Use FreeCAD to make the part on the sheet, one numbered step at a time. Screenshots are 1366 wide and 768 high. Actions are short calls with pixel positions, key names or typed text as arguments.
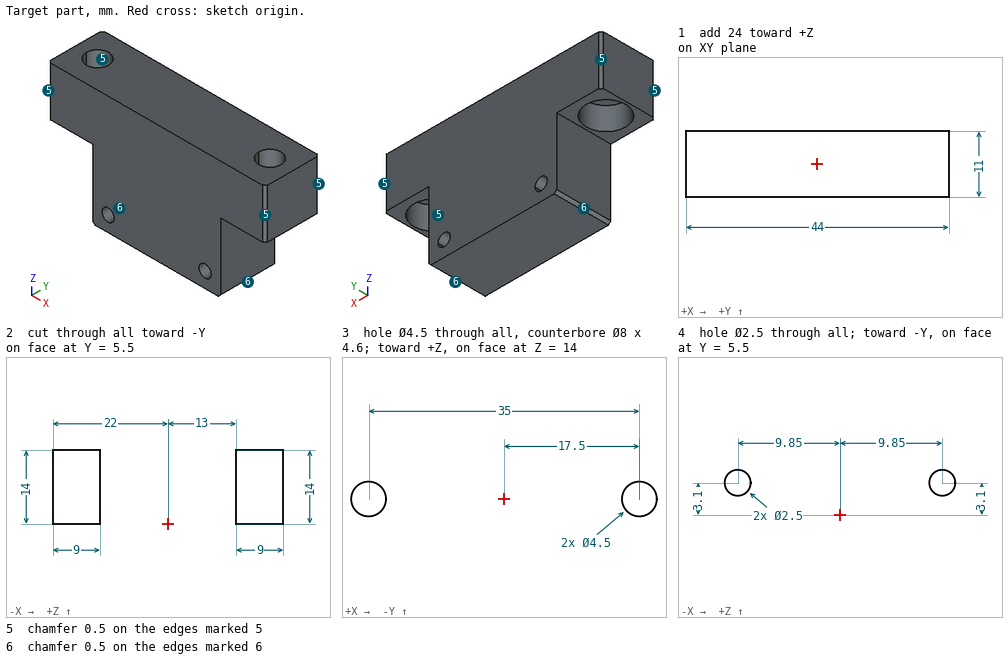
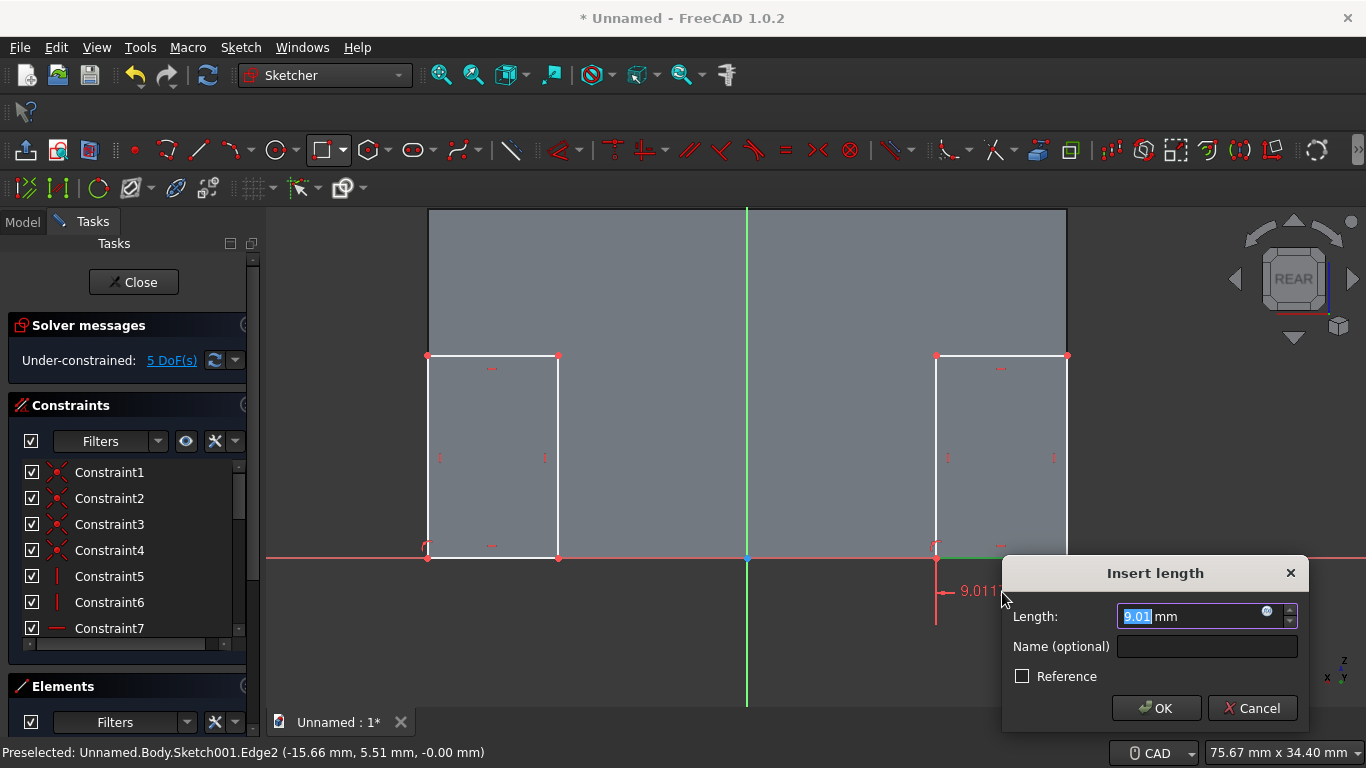
text(9)
key(Return)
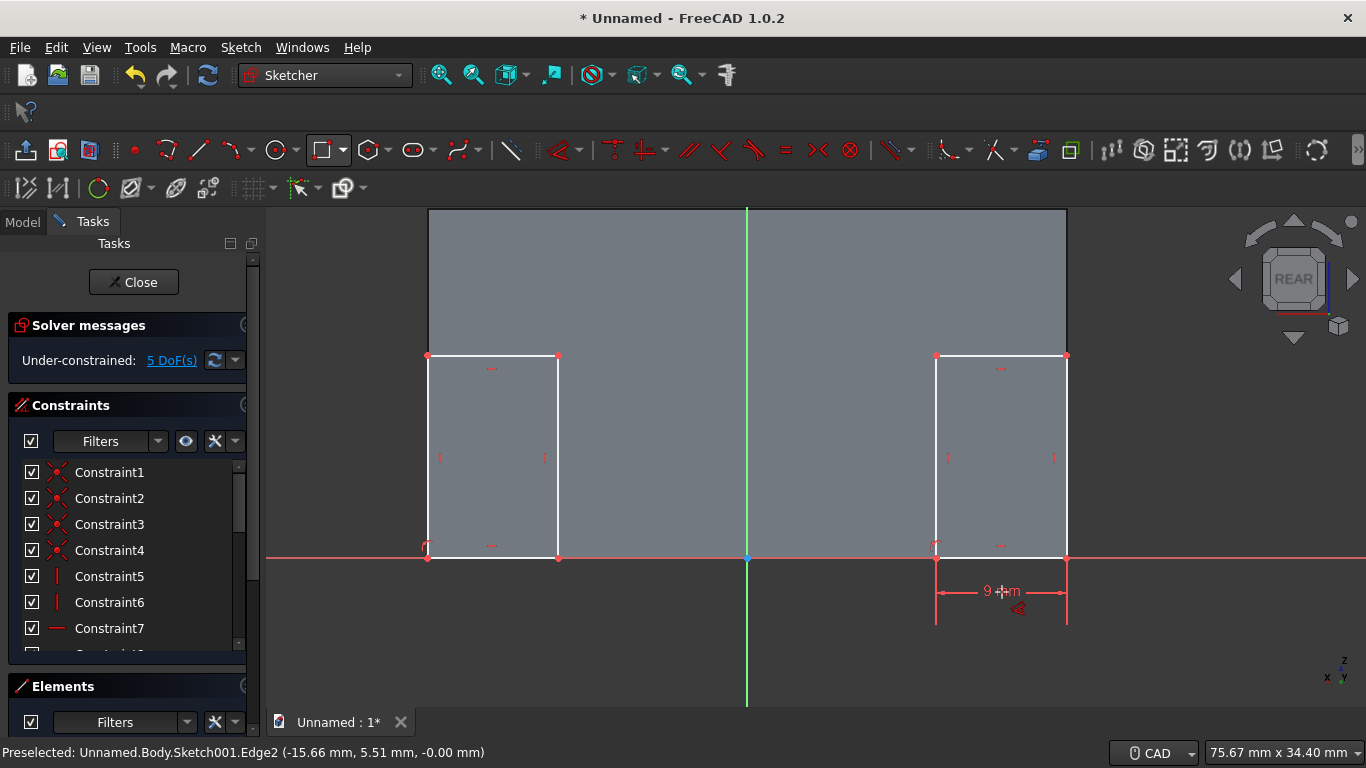
click(467, 558)
click(493, 592)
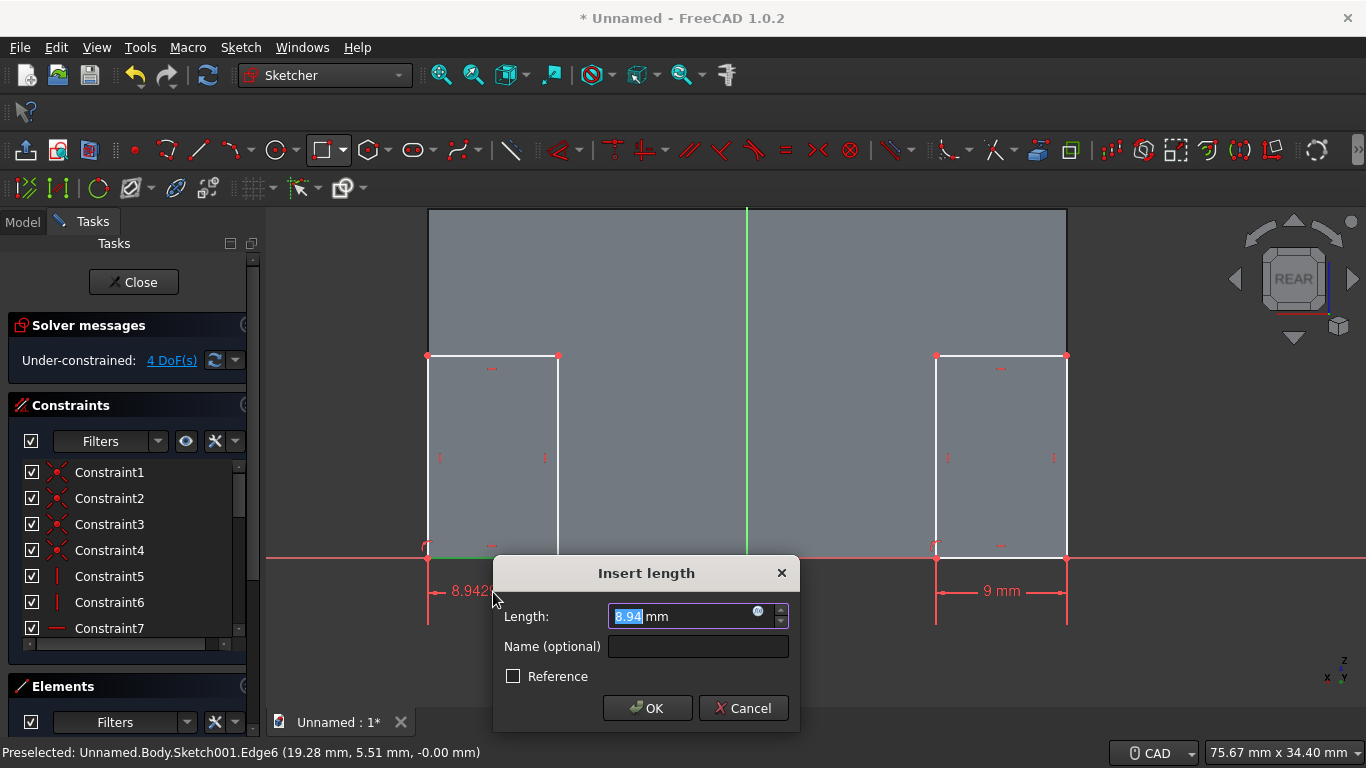
text(9)
key(Return)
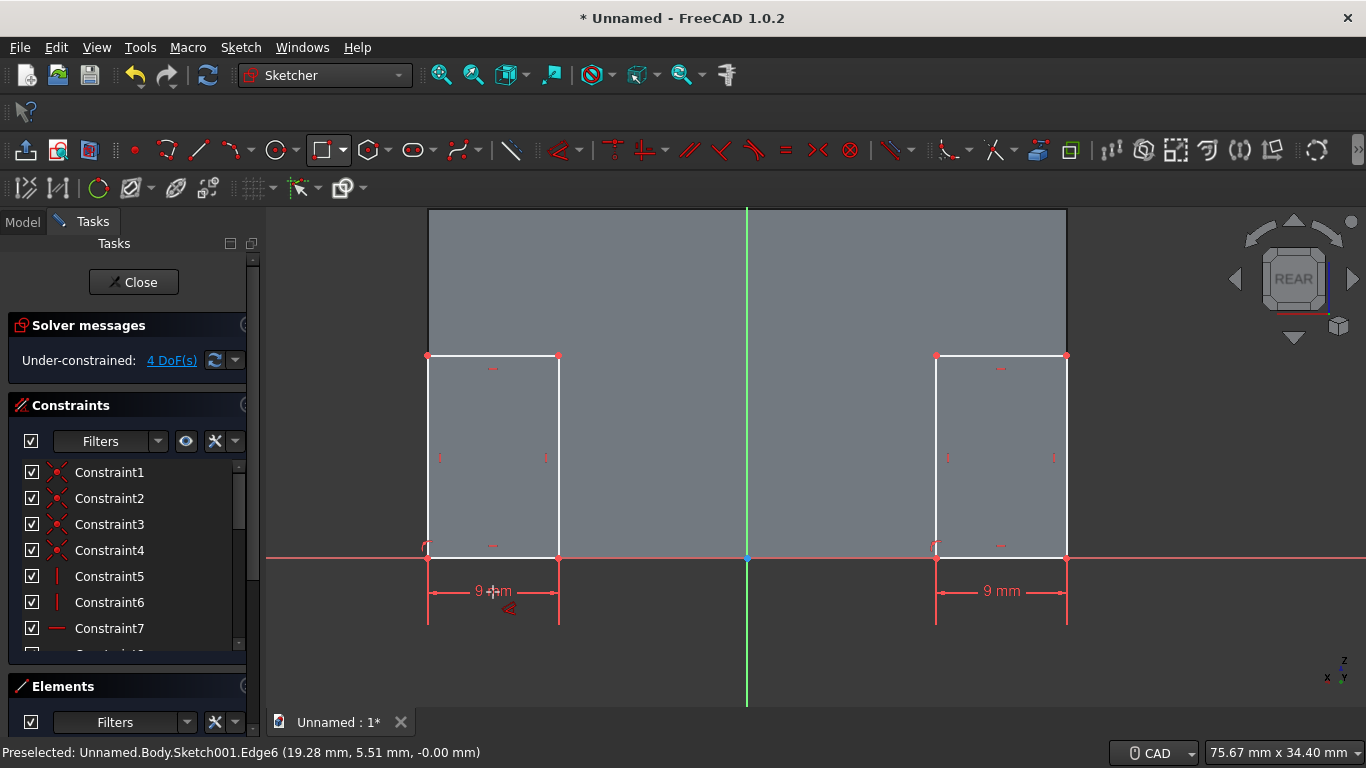
click(936, 417)
click(970, 457)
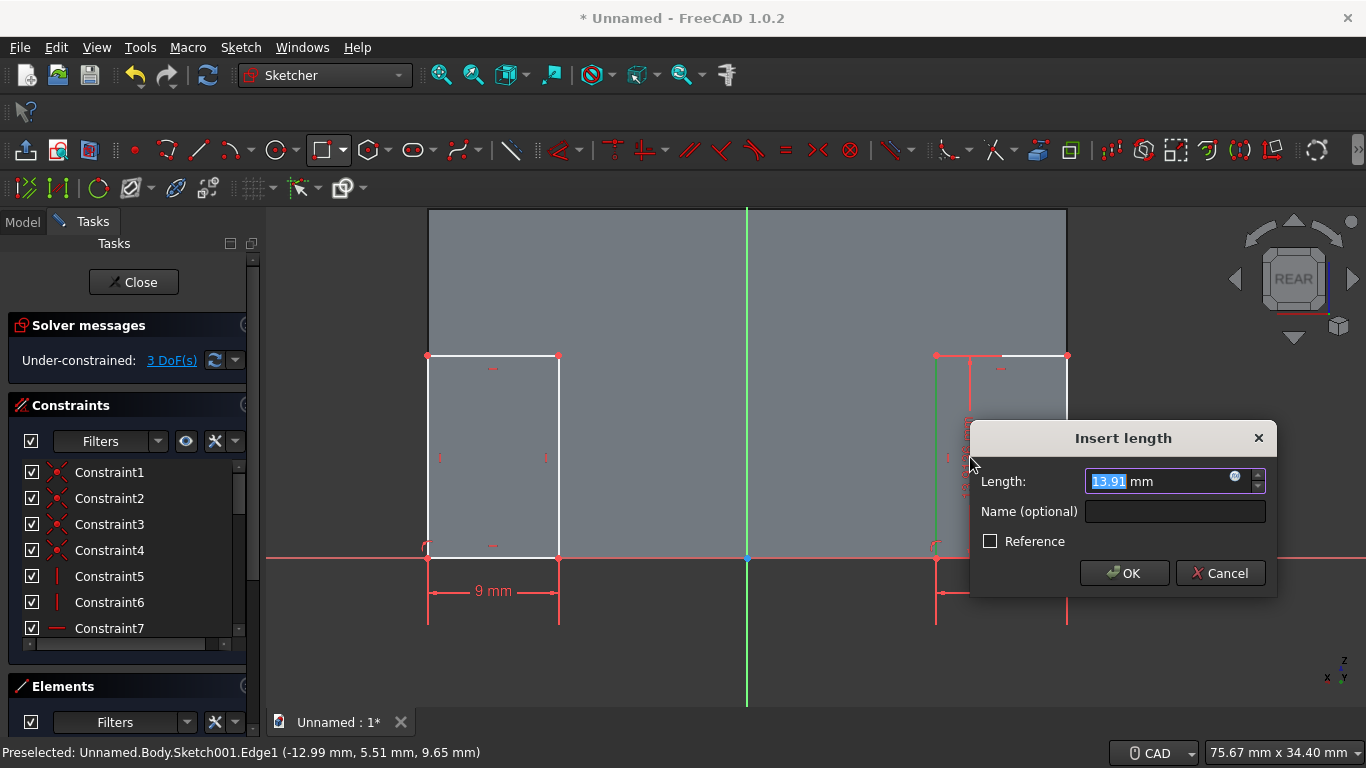
text(14)
key(Return)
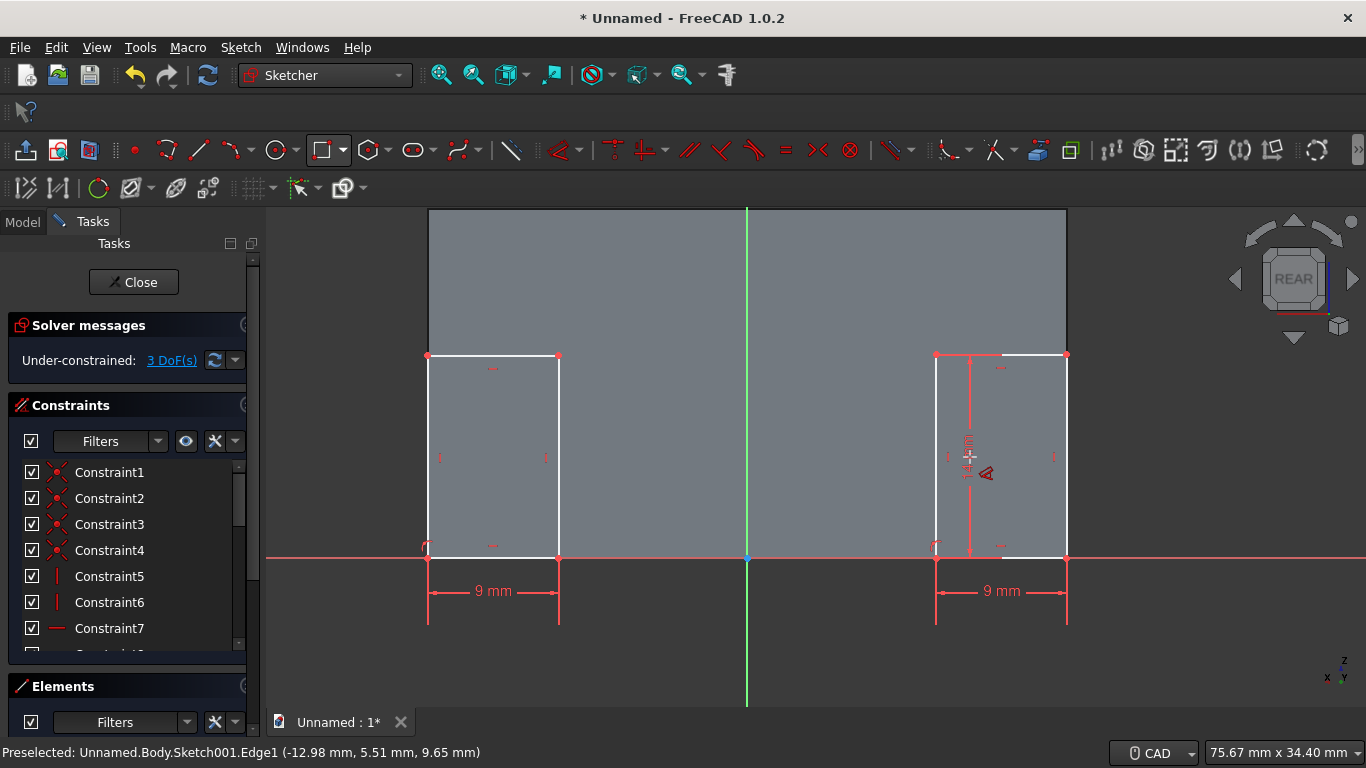
click(428, 417)
click(394, 457)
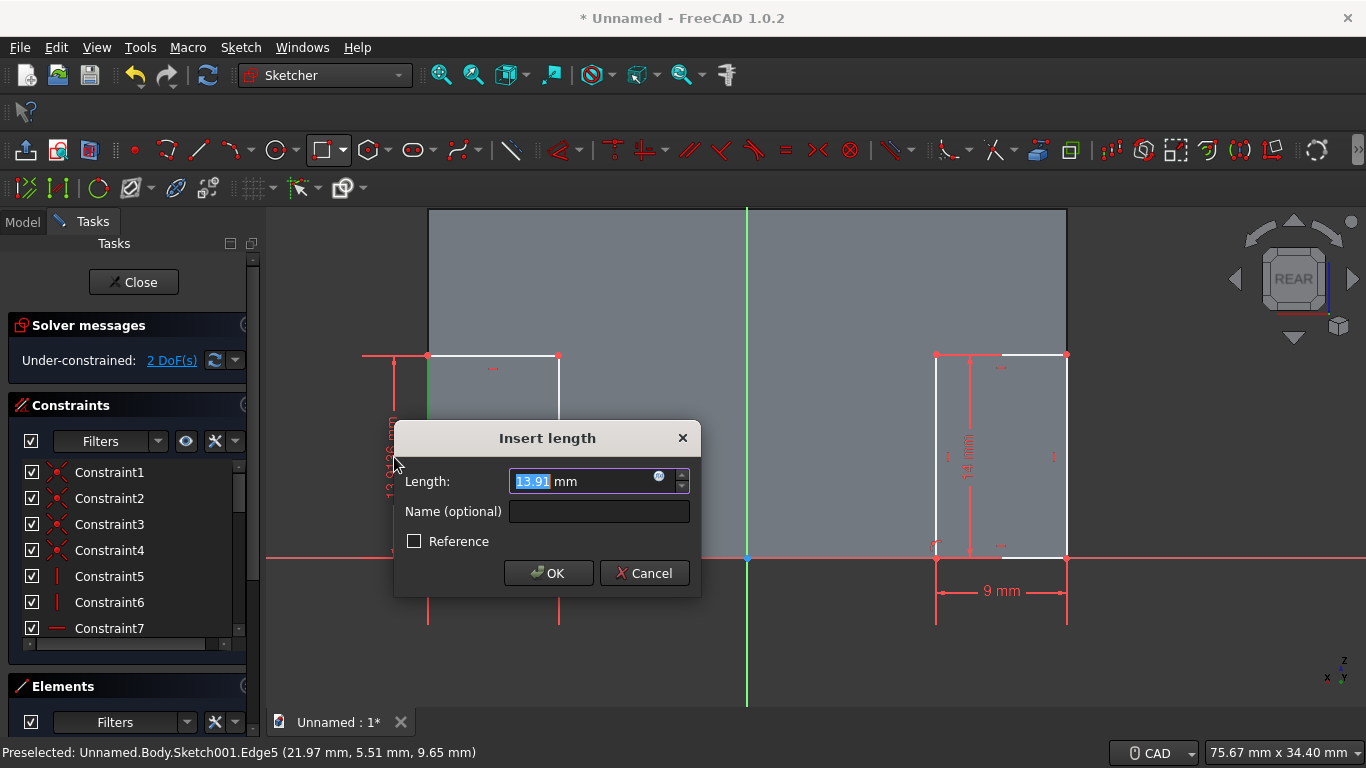
text(14)
key(Return)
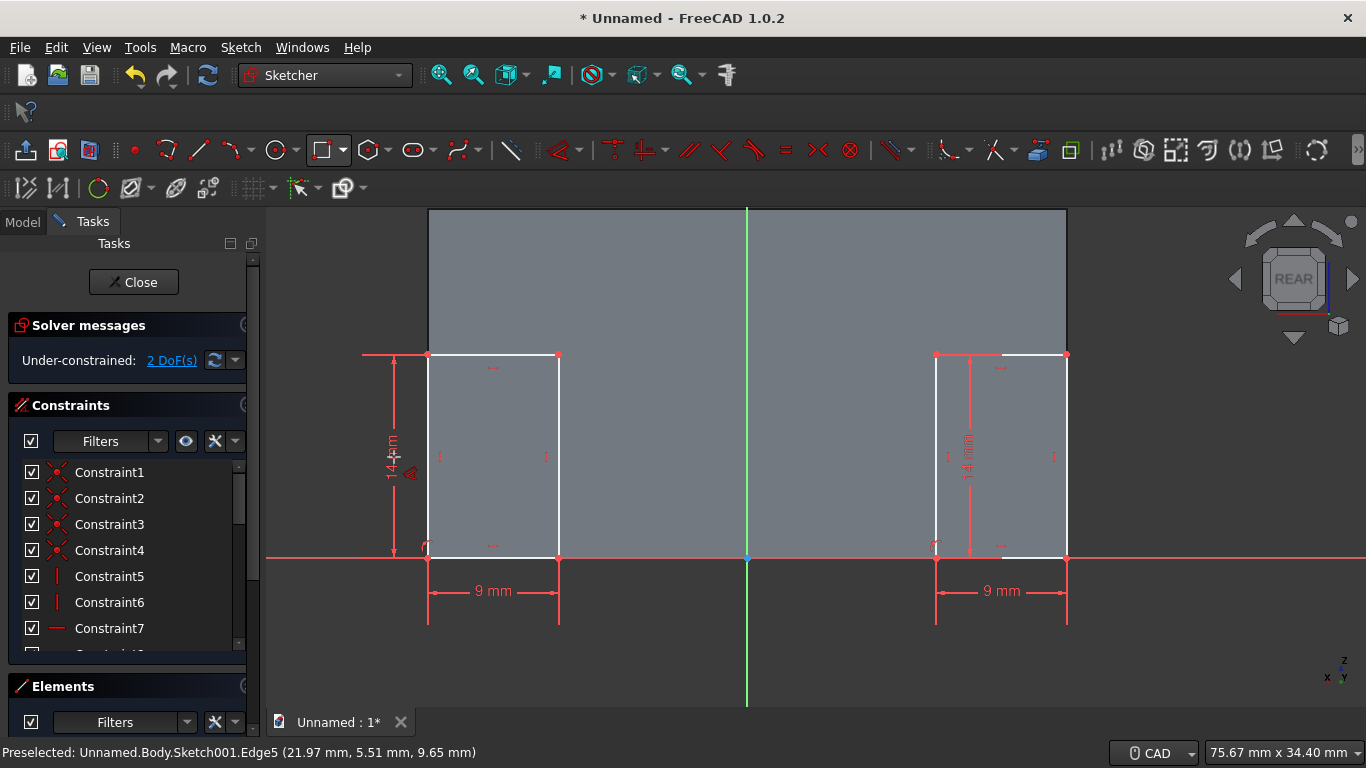
click(936, 355)
click(842, 592)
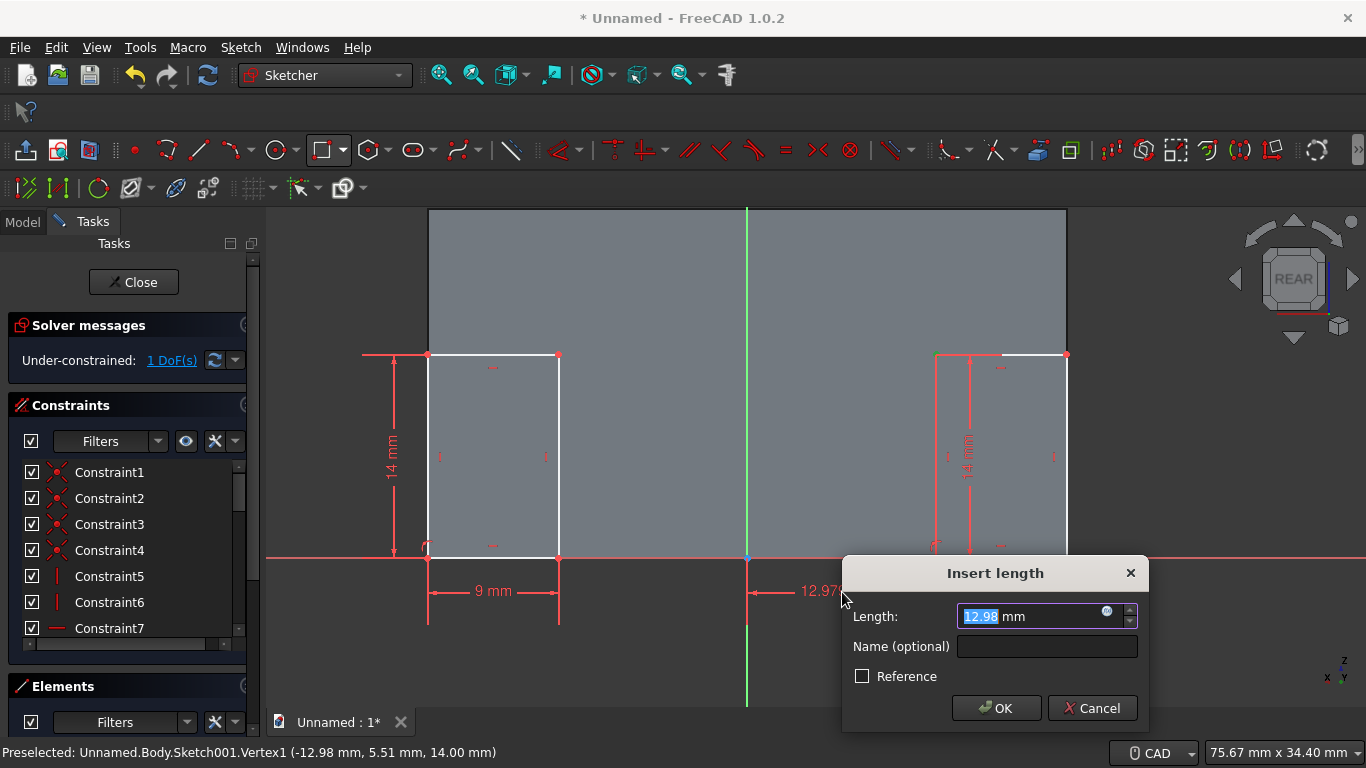
text(13)
key(Return)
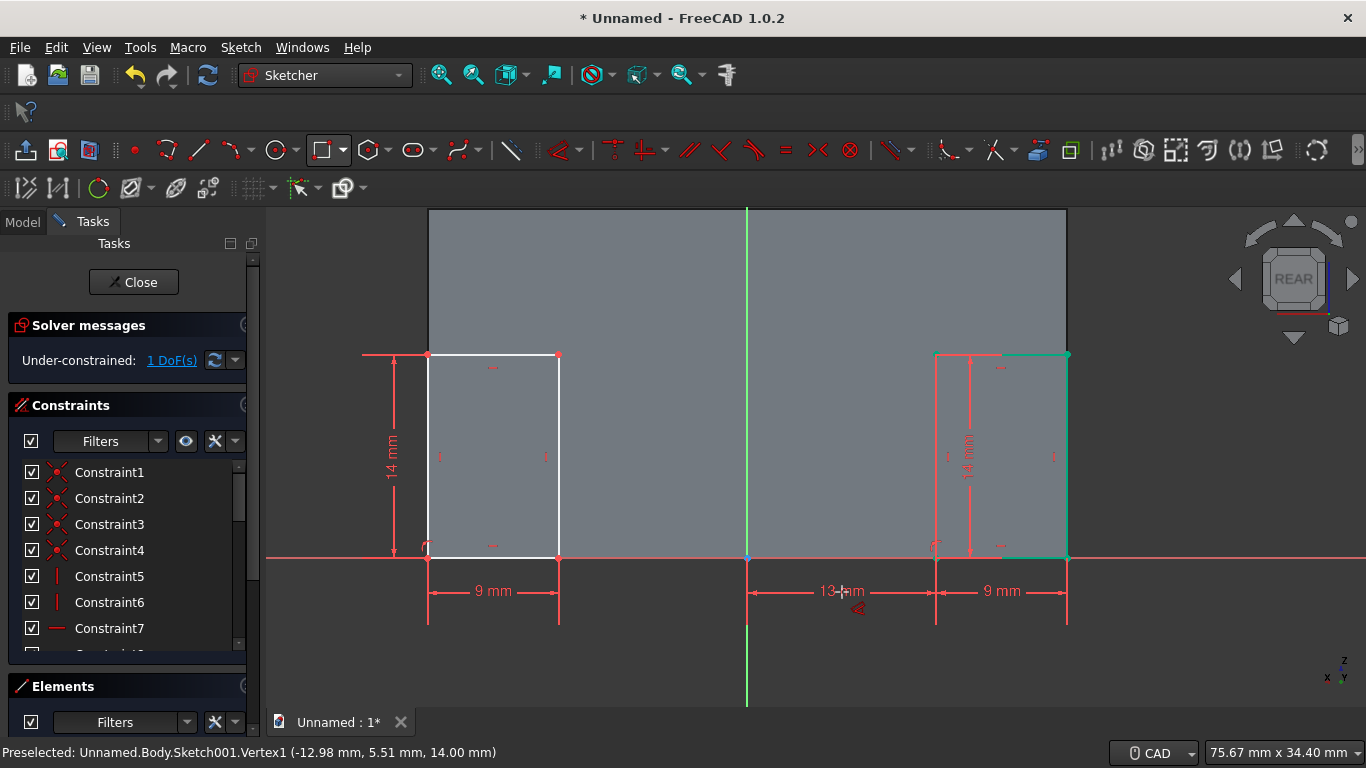
click(428, 355)
click(588, 592)